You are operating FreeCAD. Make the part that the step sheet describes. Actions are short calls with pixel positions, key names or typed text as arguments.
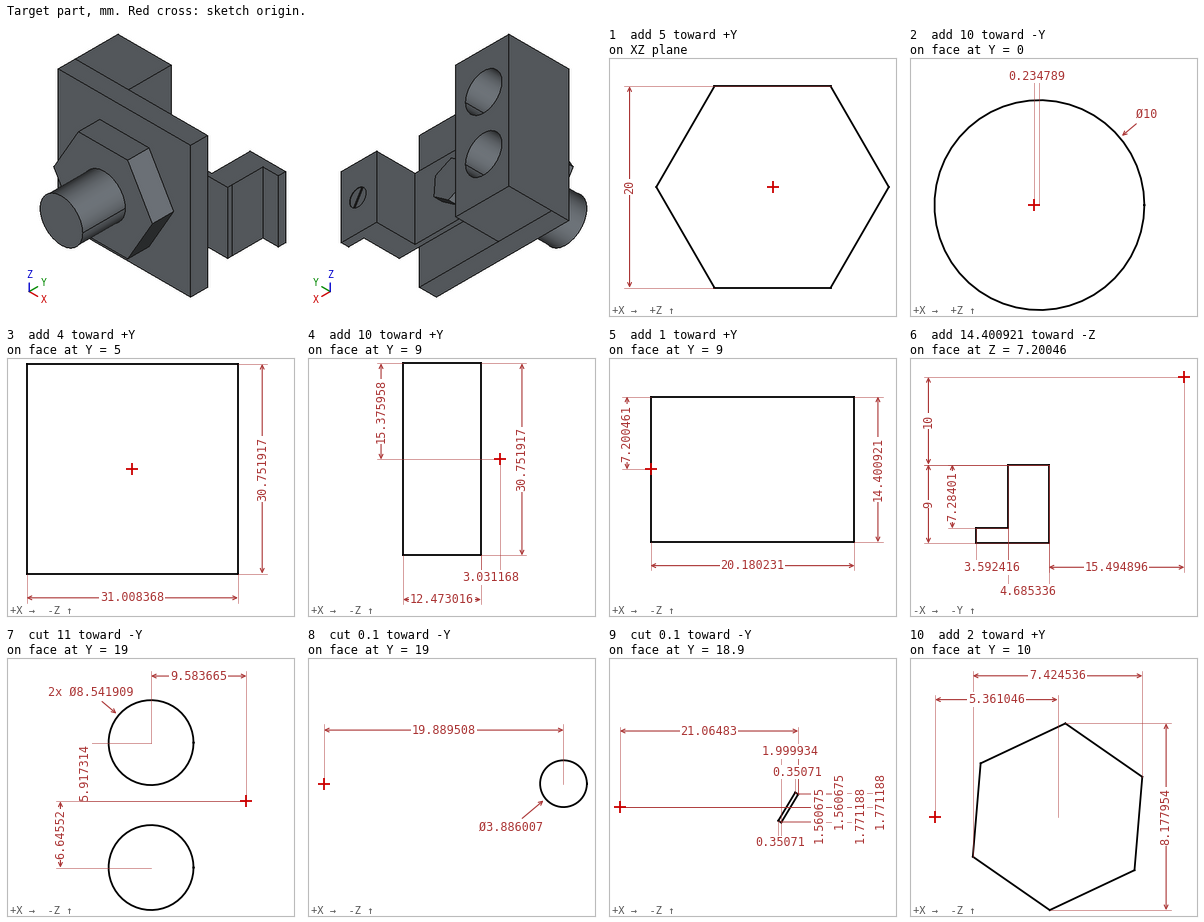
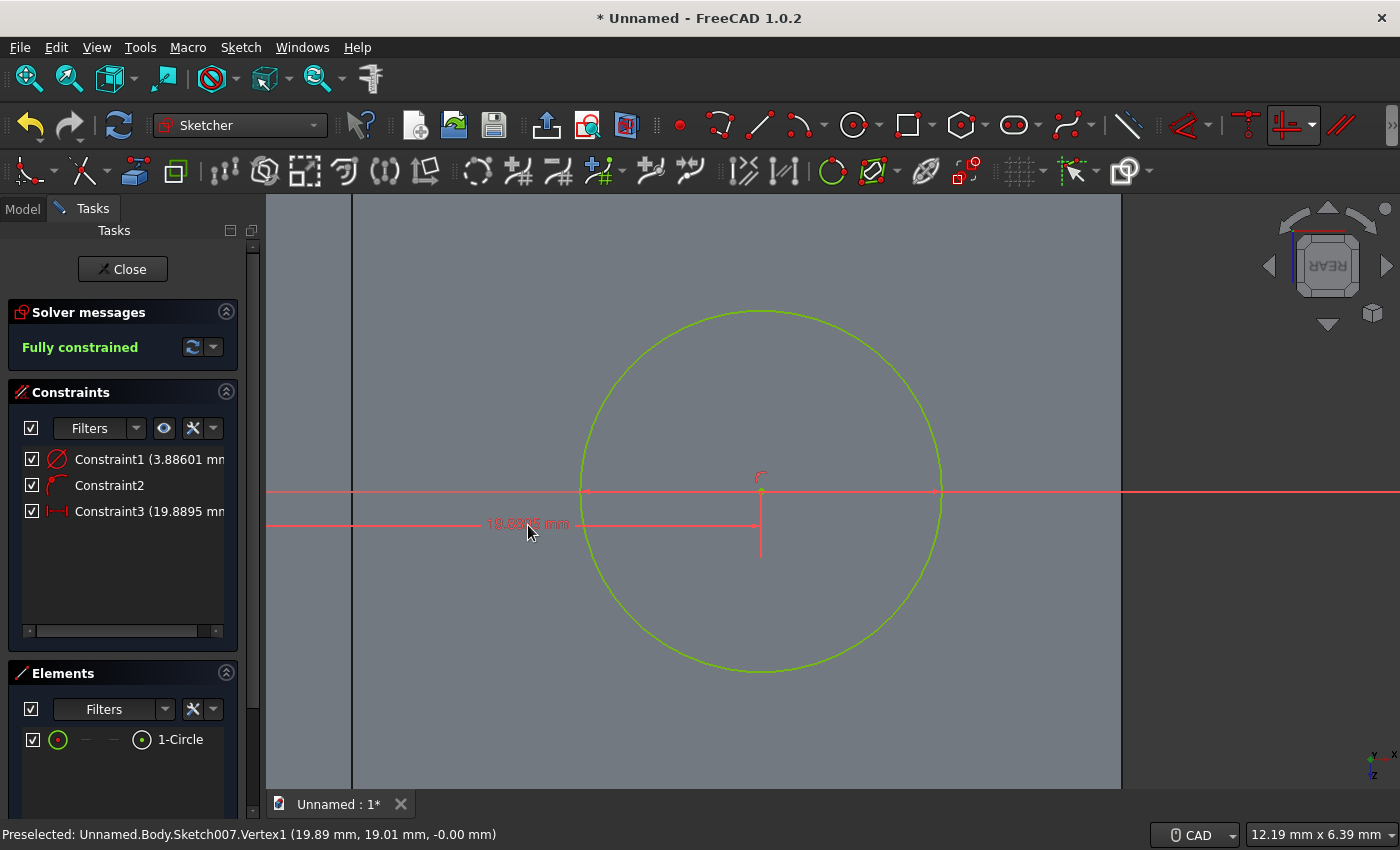
click(123, 269)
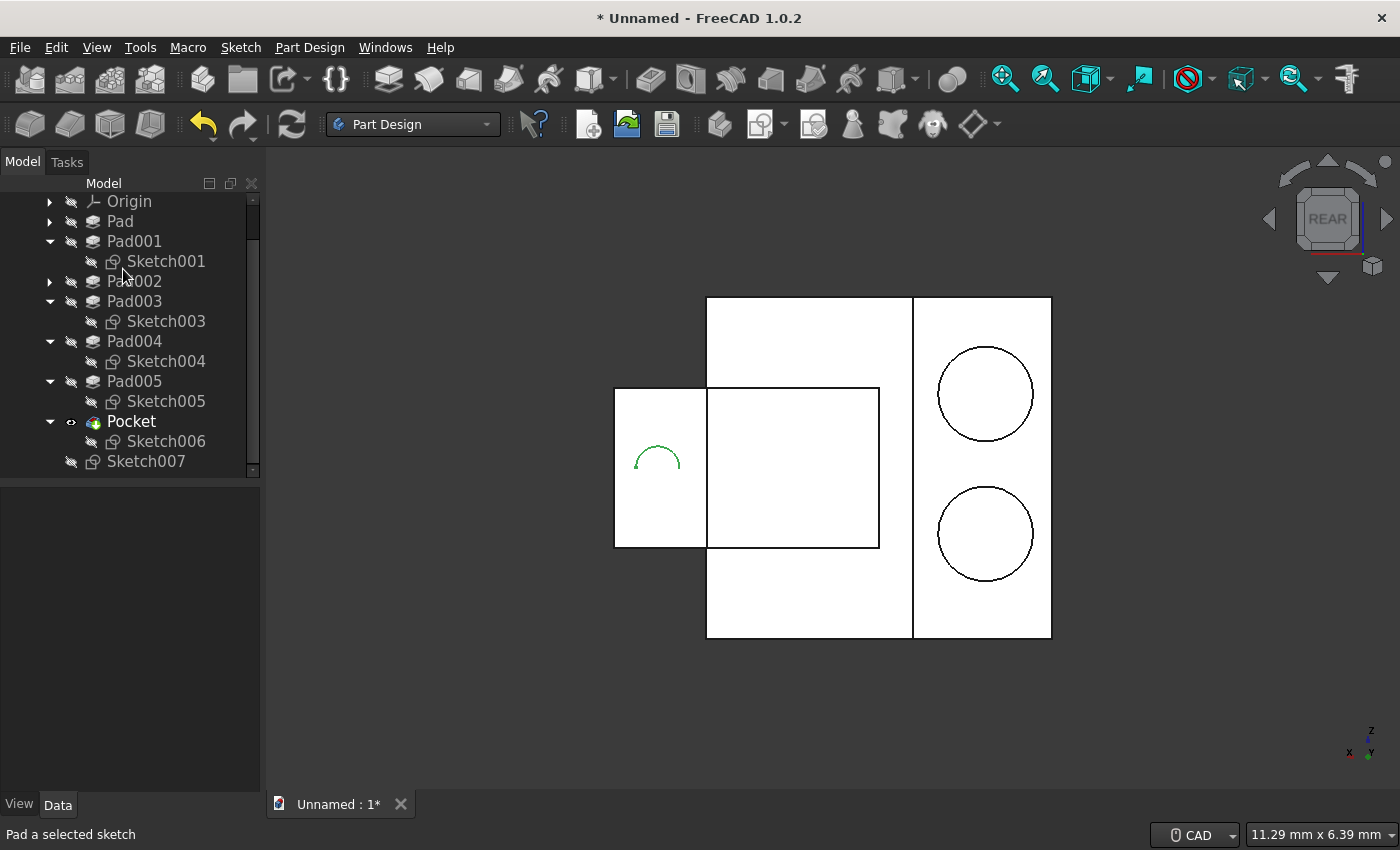
click(652, 80)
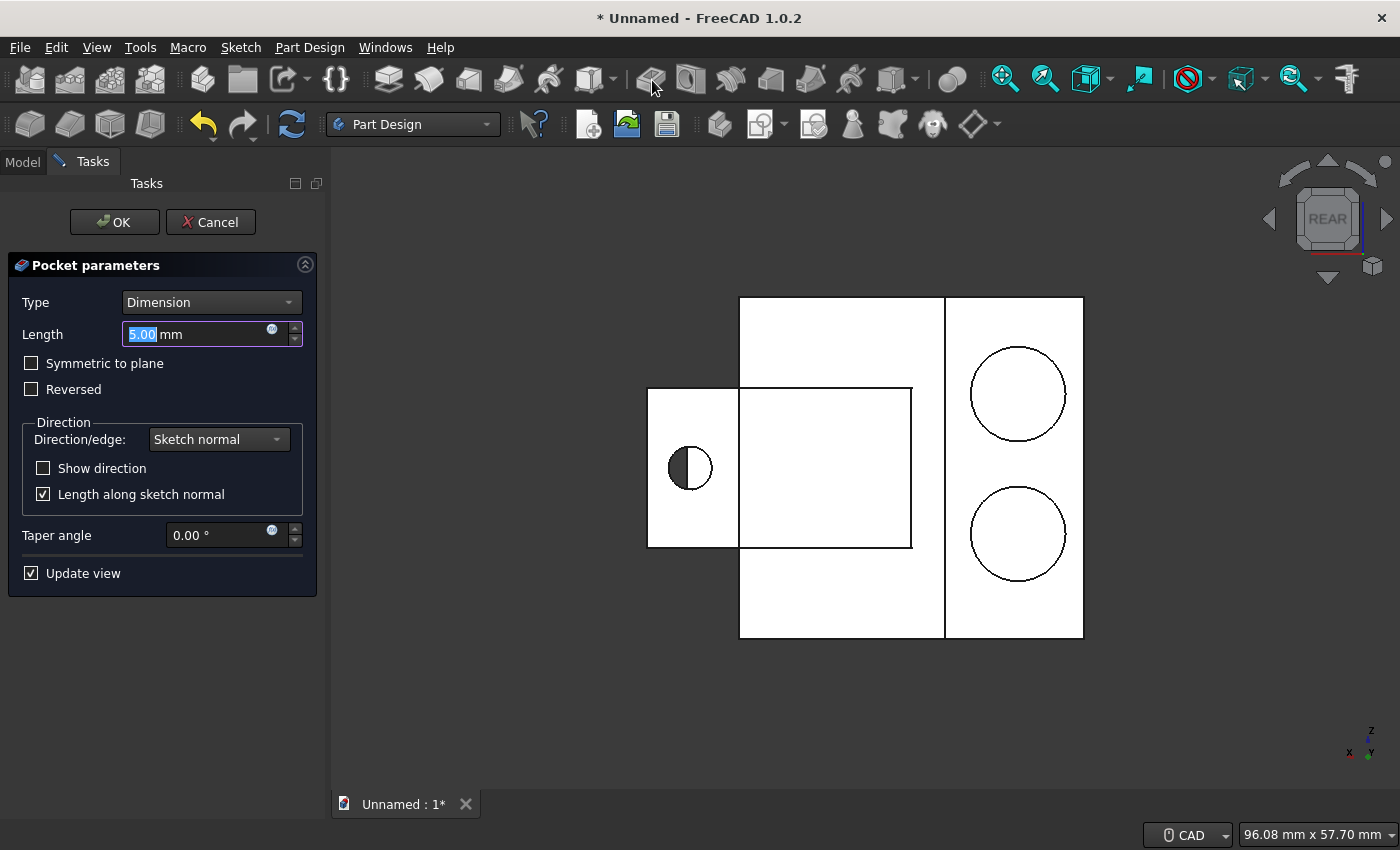
text(0.1)
key(Tab)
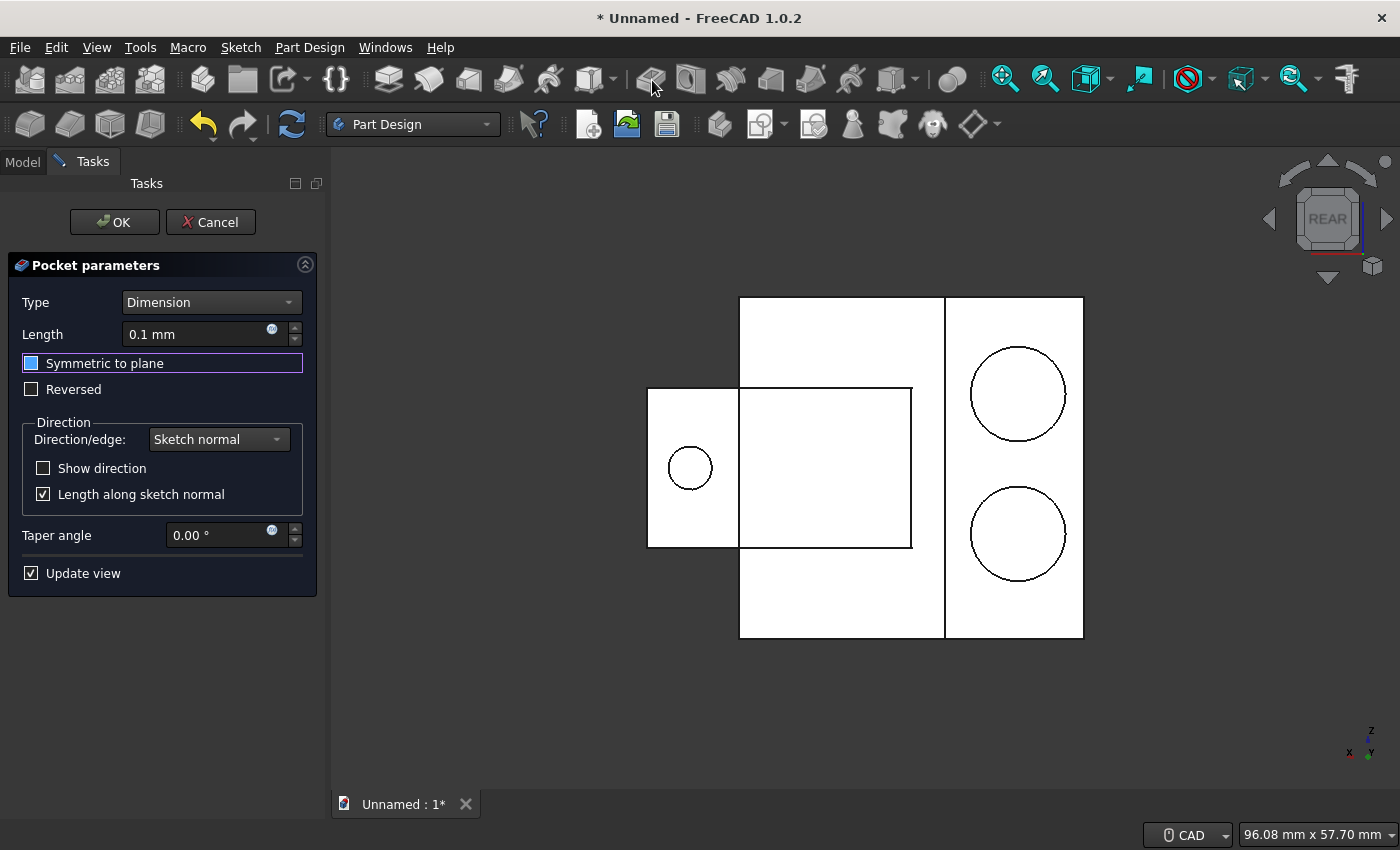
click(115, 222)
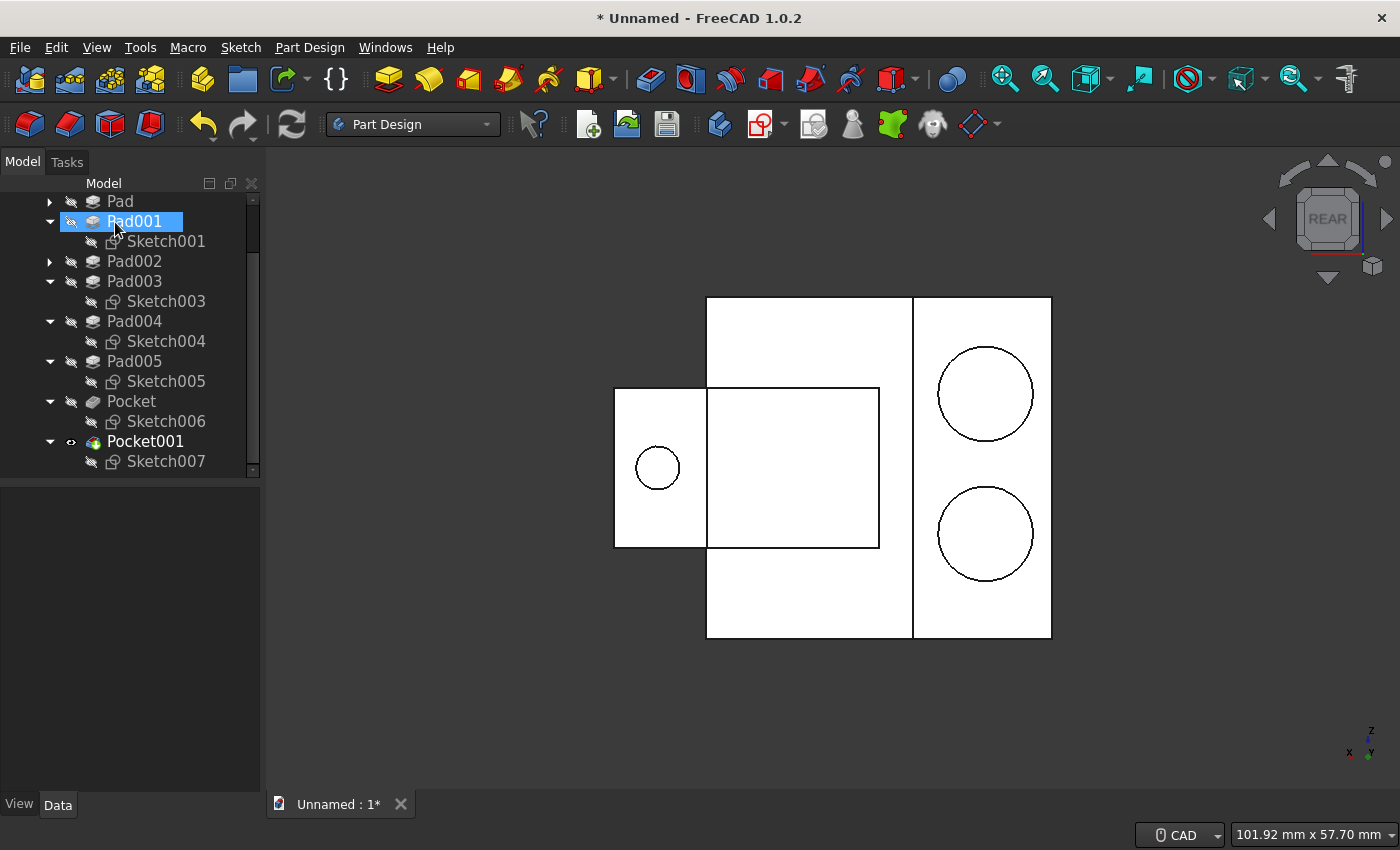
click(658, 467)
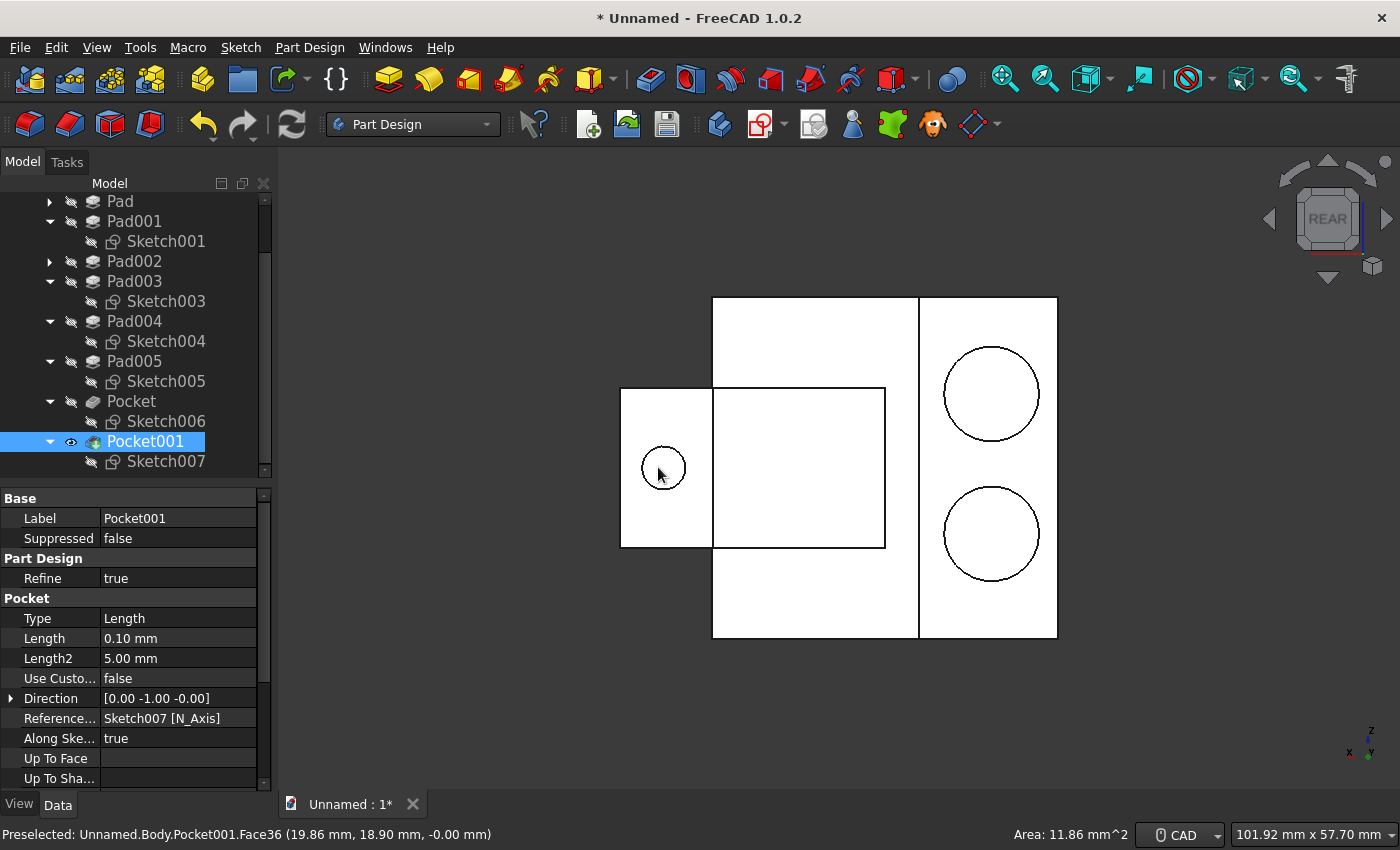
click(760, 124)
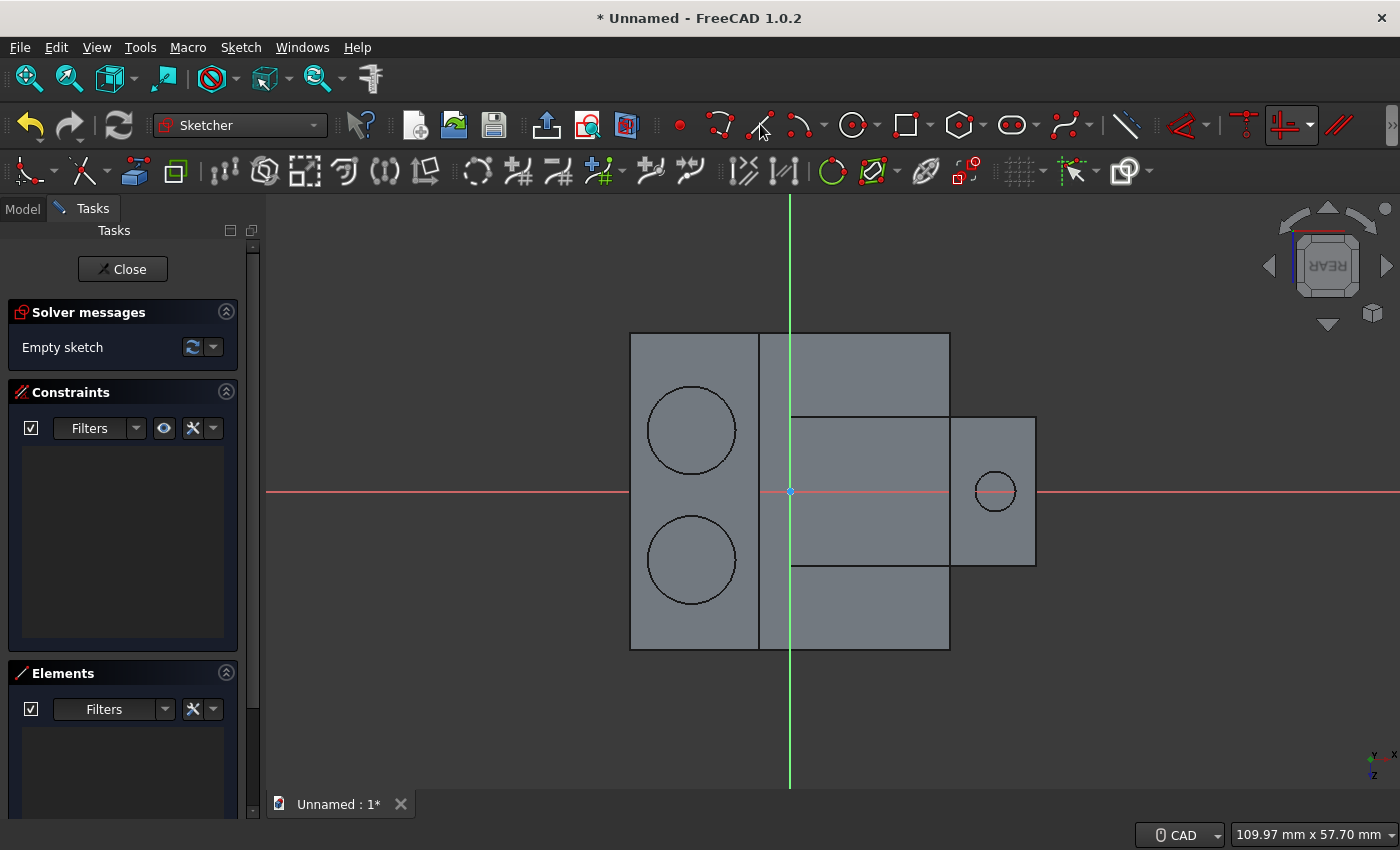
click(628, 126)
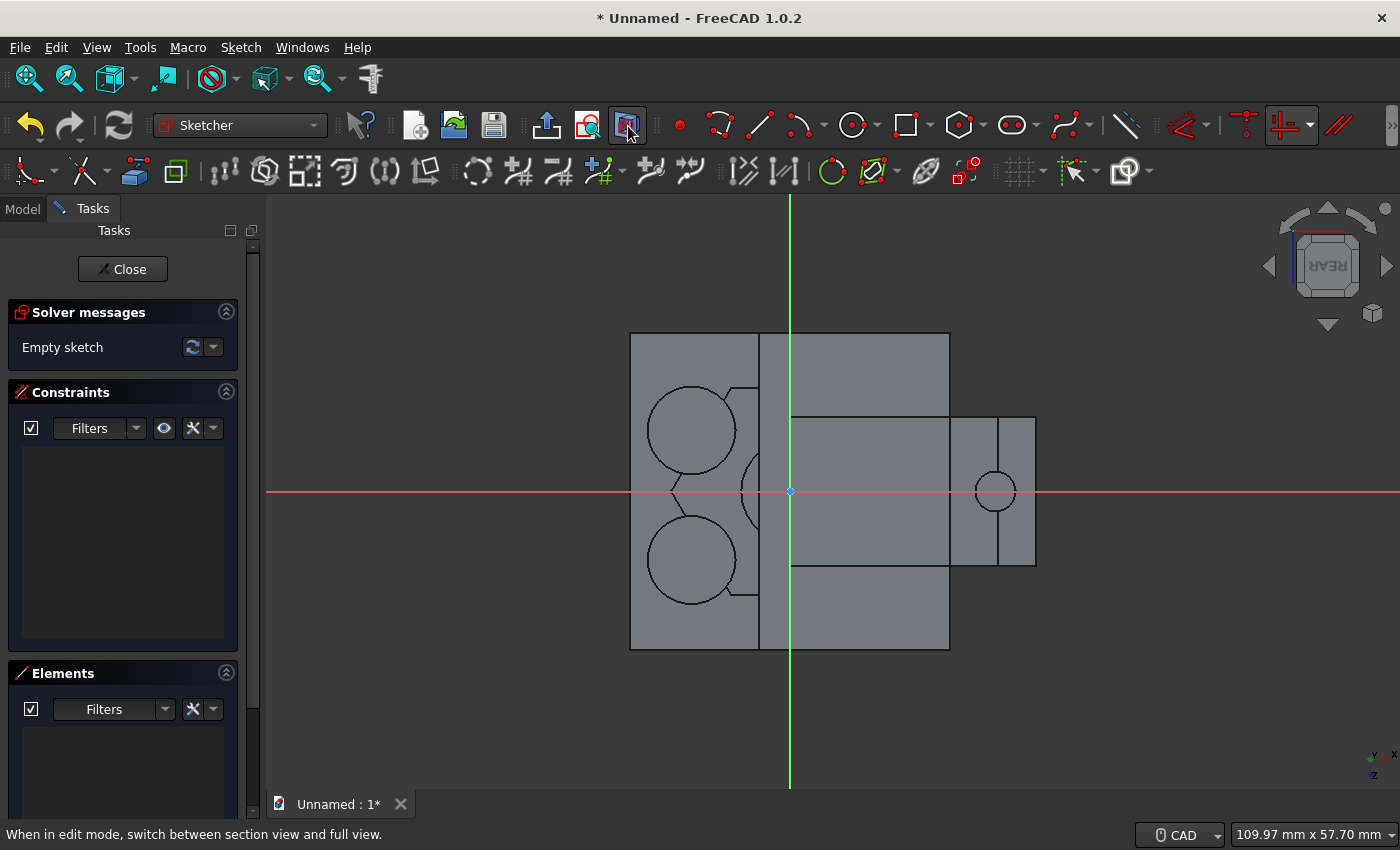
scroll(1019, 491, up, 12)